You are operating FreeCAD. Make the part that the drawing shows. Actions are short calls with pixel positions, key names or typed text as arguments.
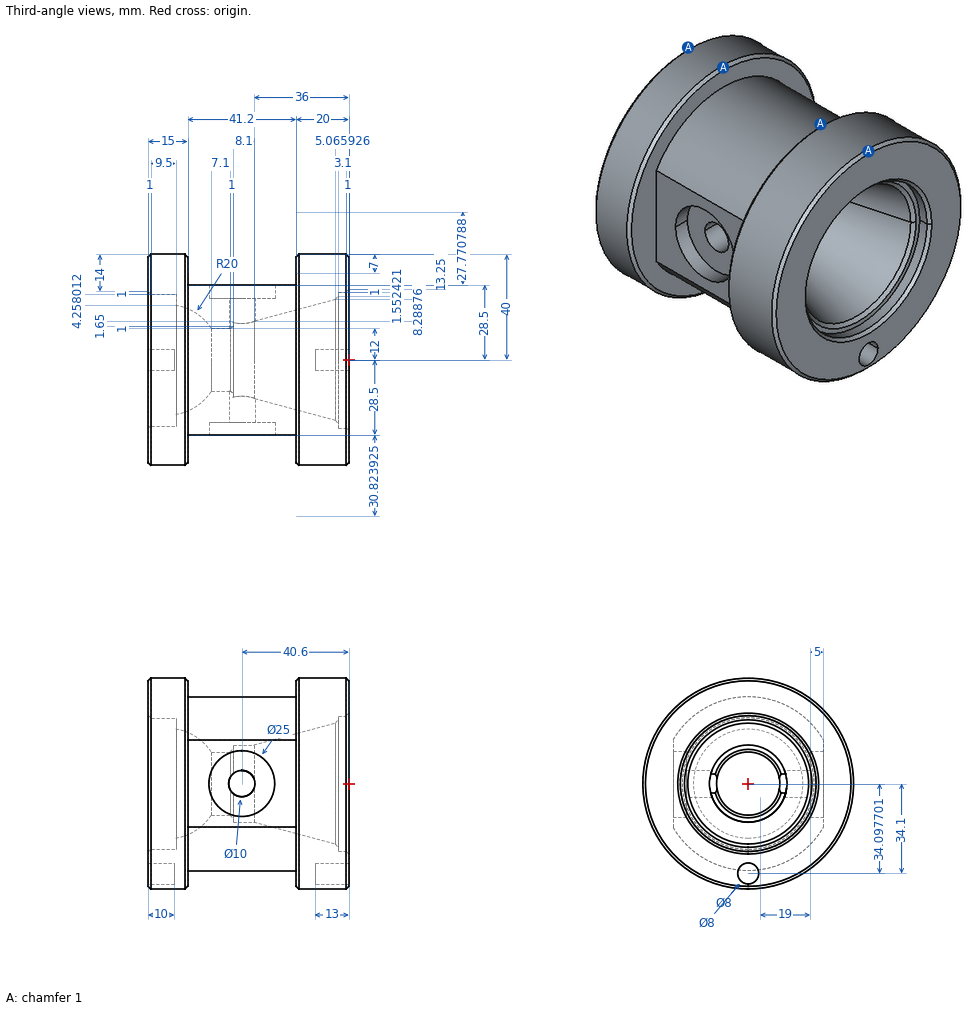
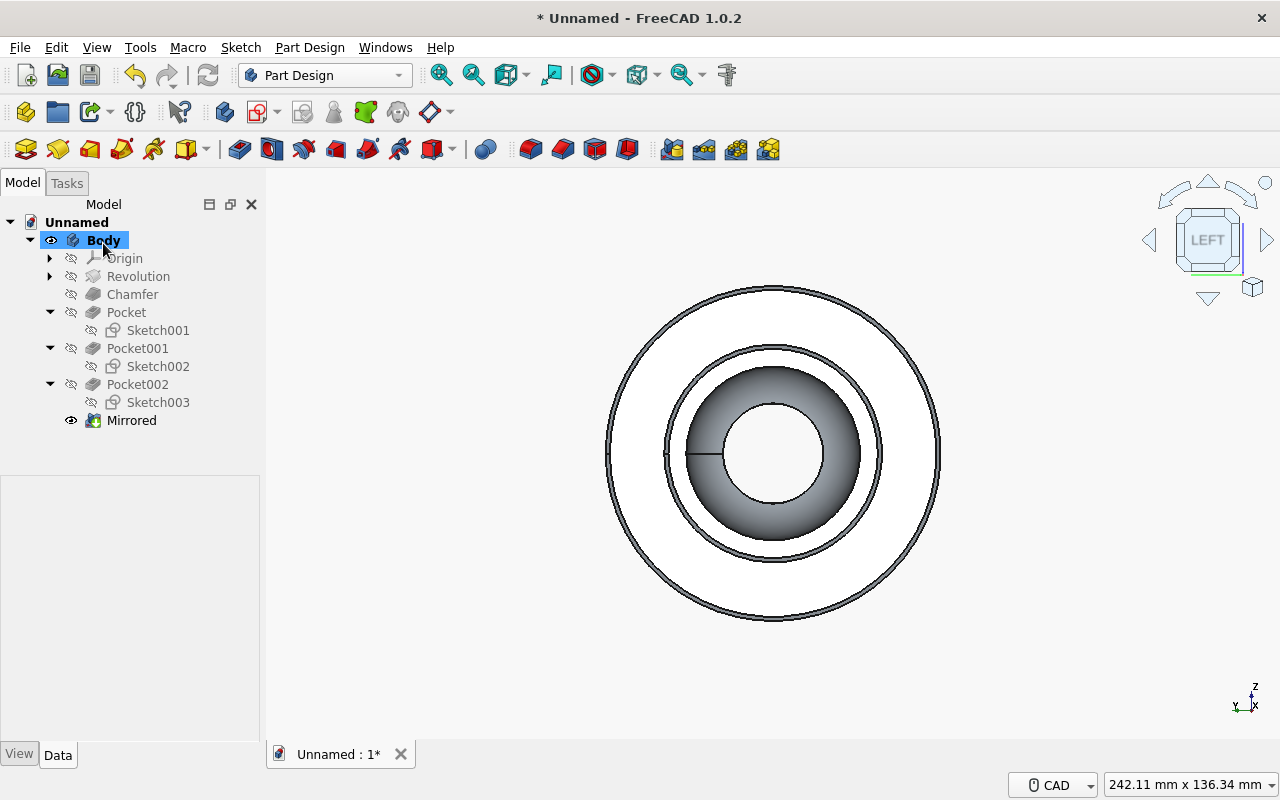
click(633, 453)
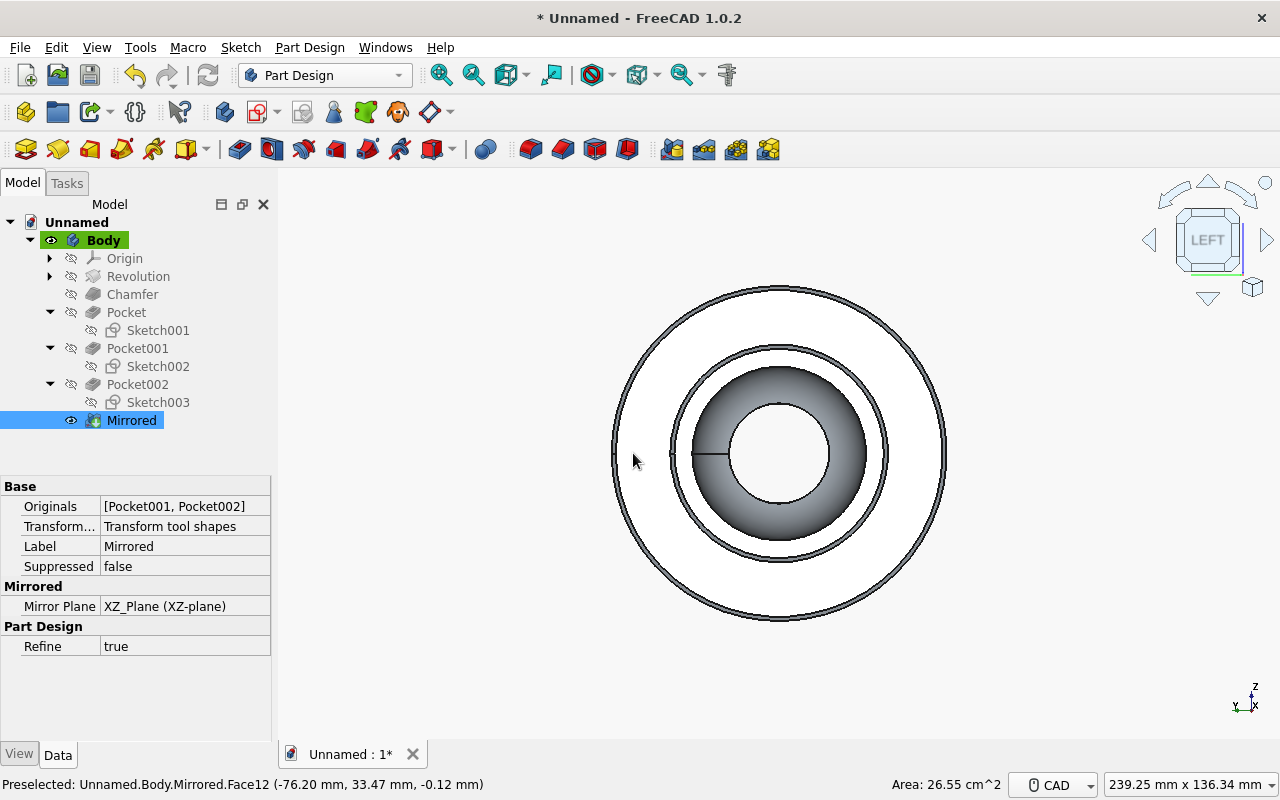
click(258, 112)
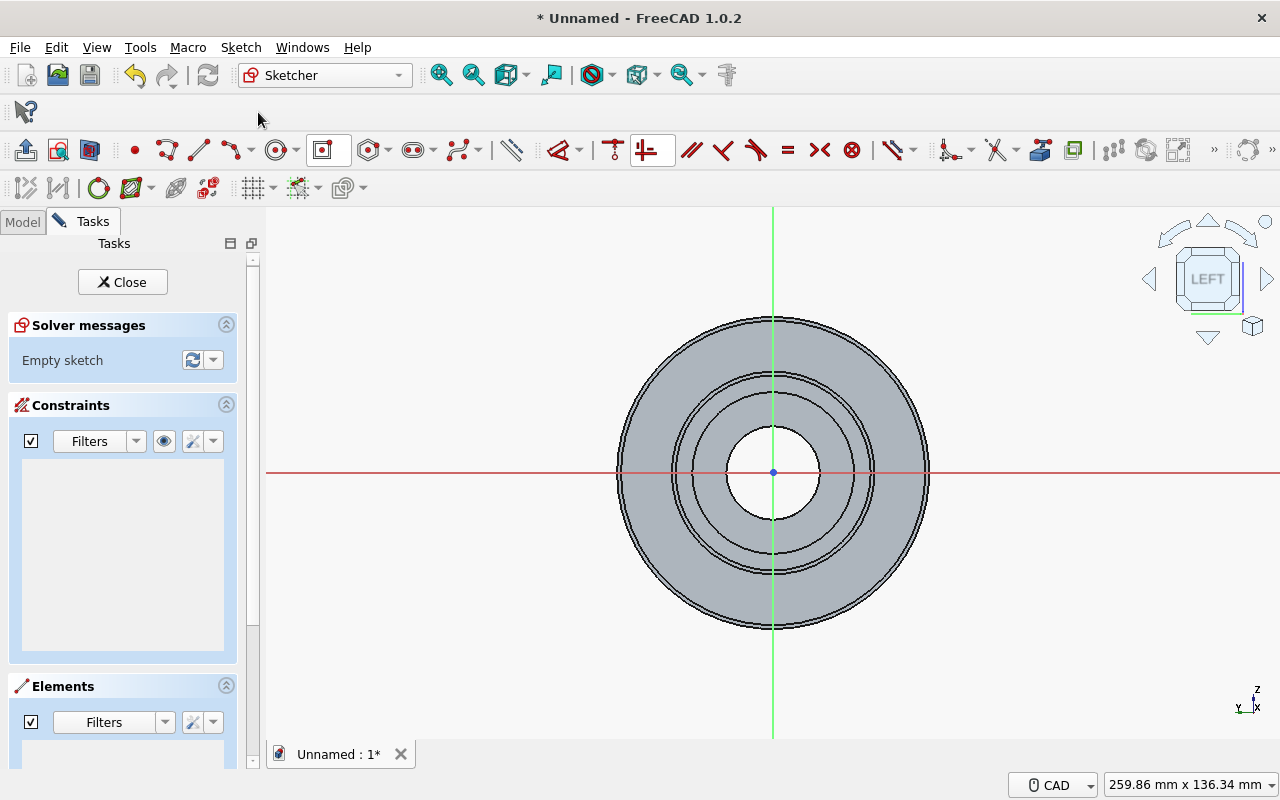
scroll(780, 619, up, 12)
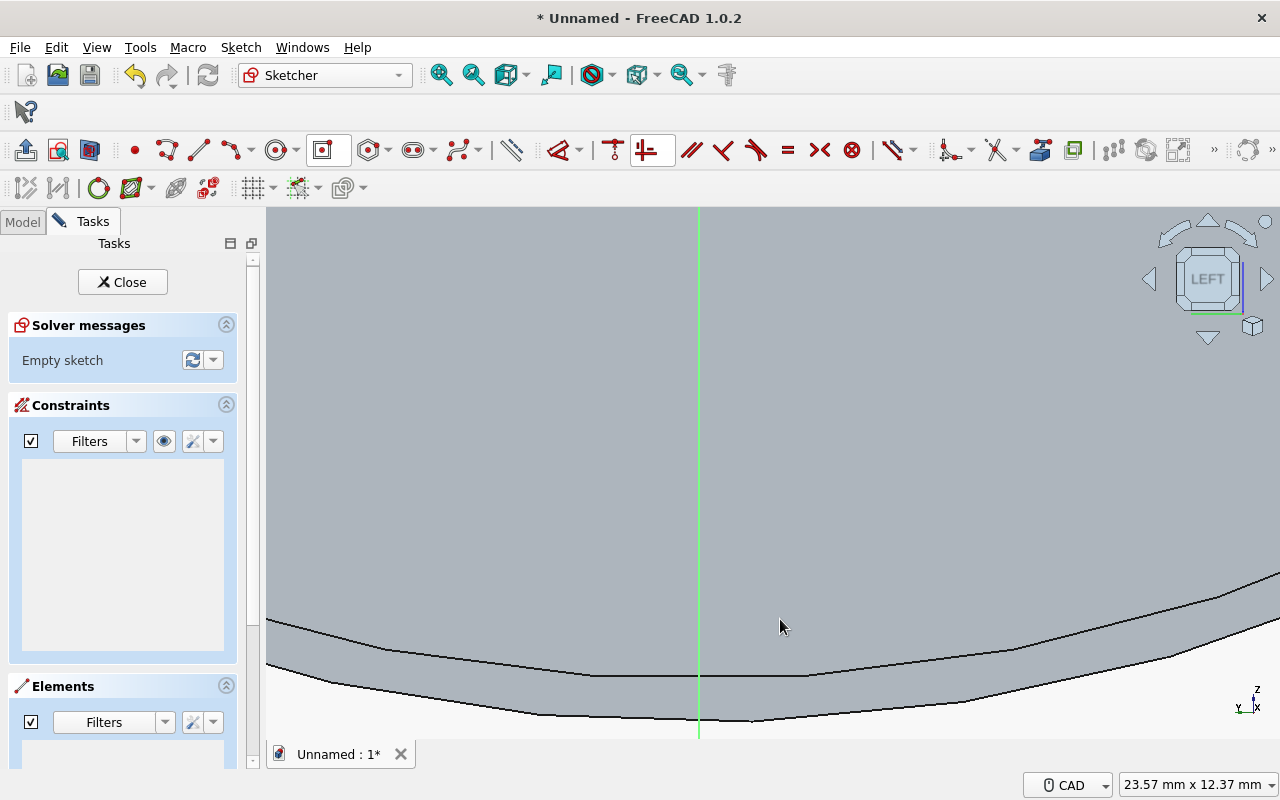
click(276, 150)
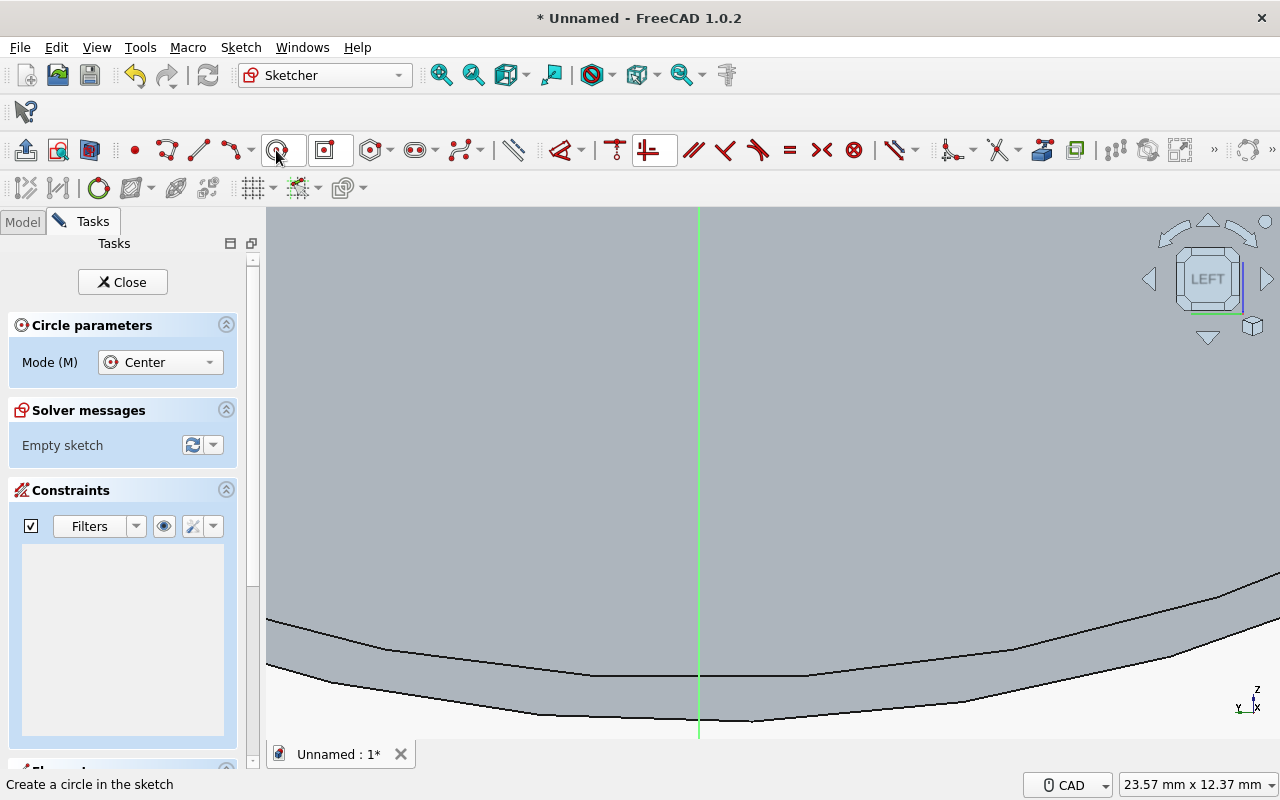
click(699, 468)
move(821, 347)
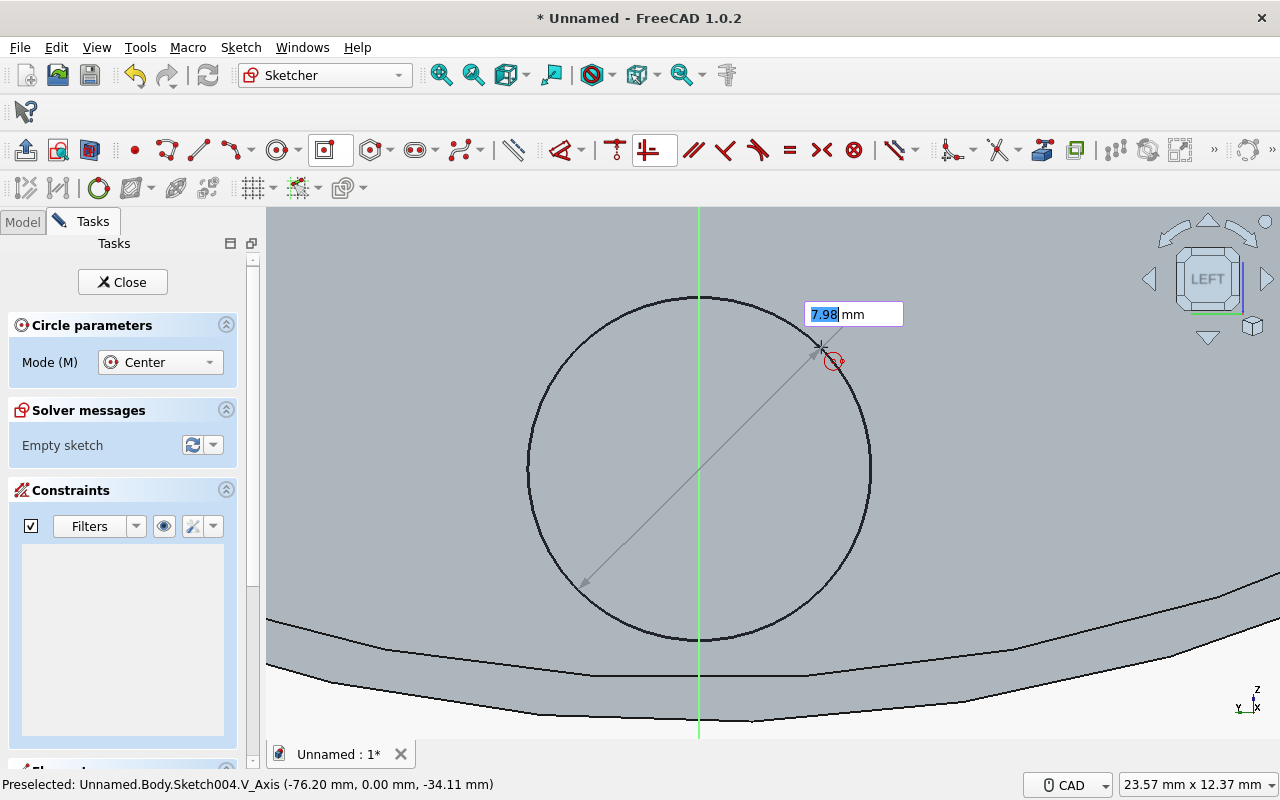
text(8)
key(Return)
key(Escape)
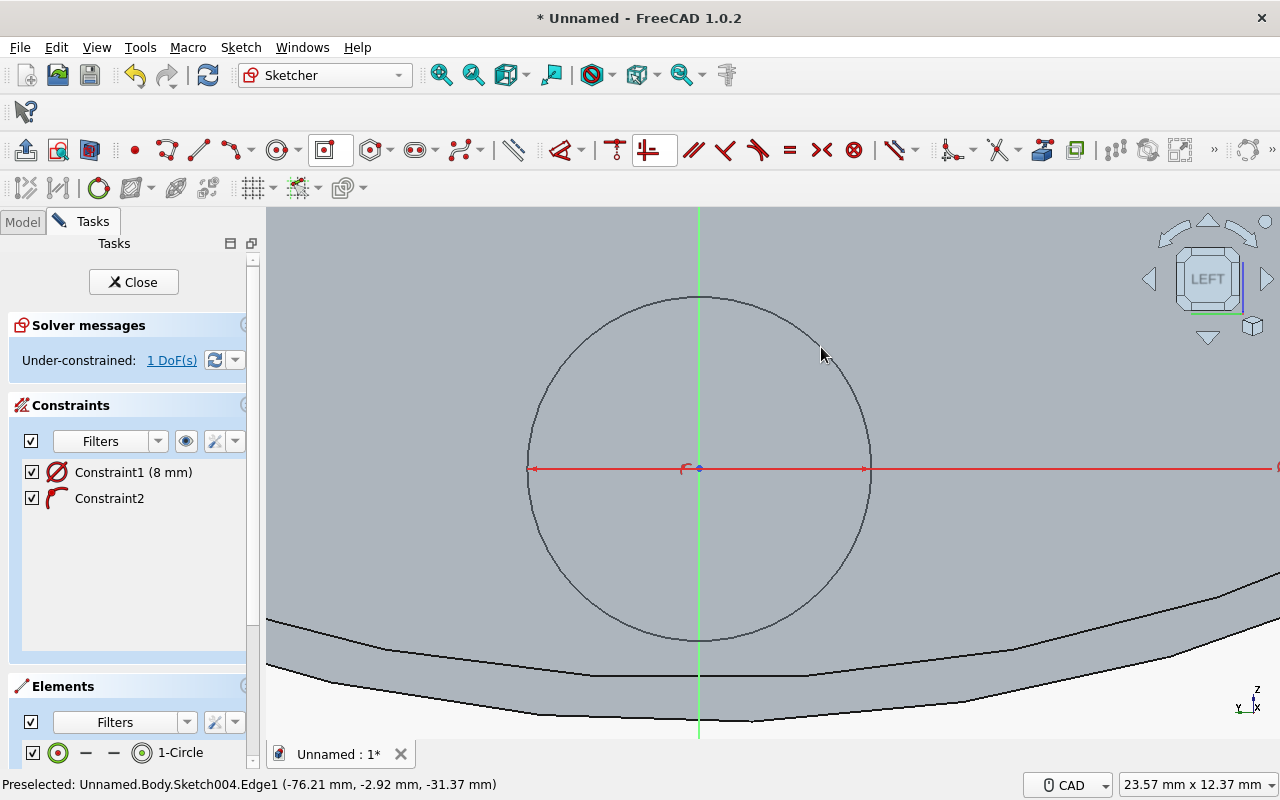
click(560, 150)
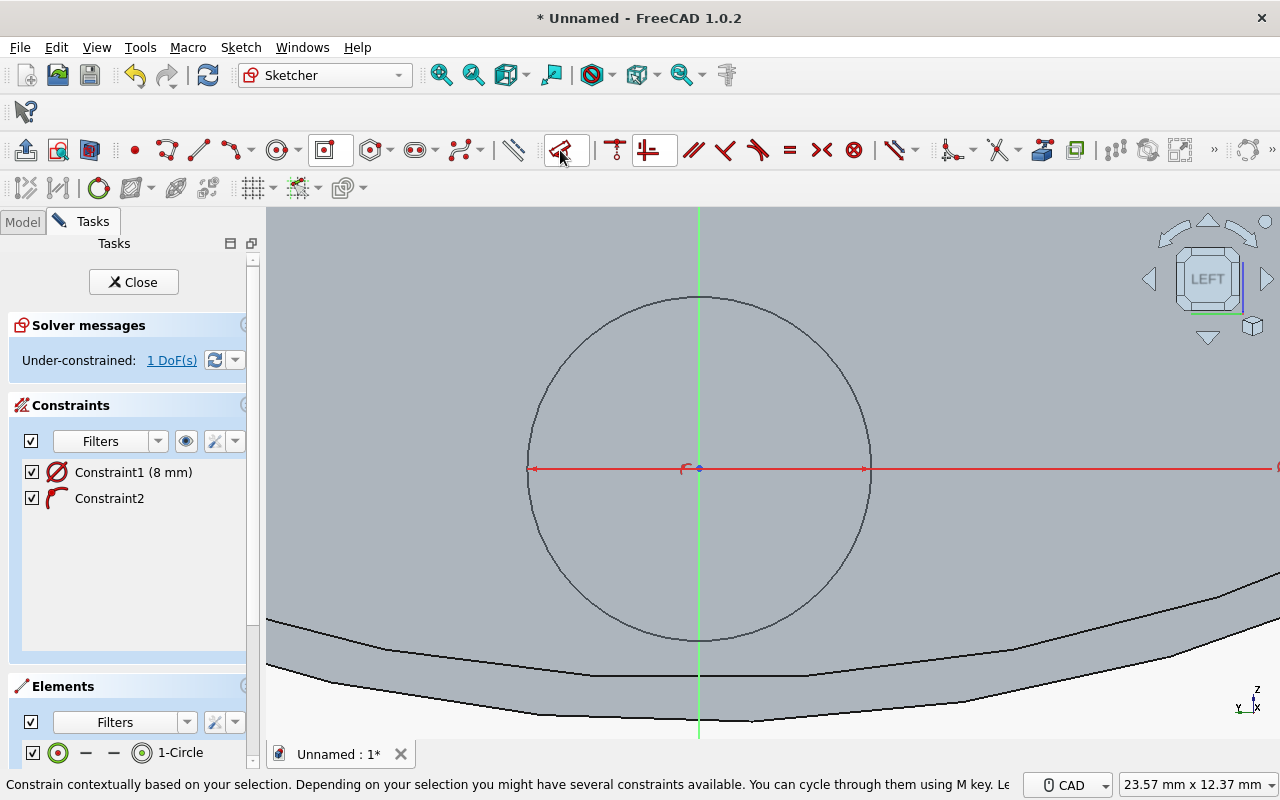
click(699, 469)
click(733, 352)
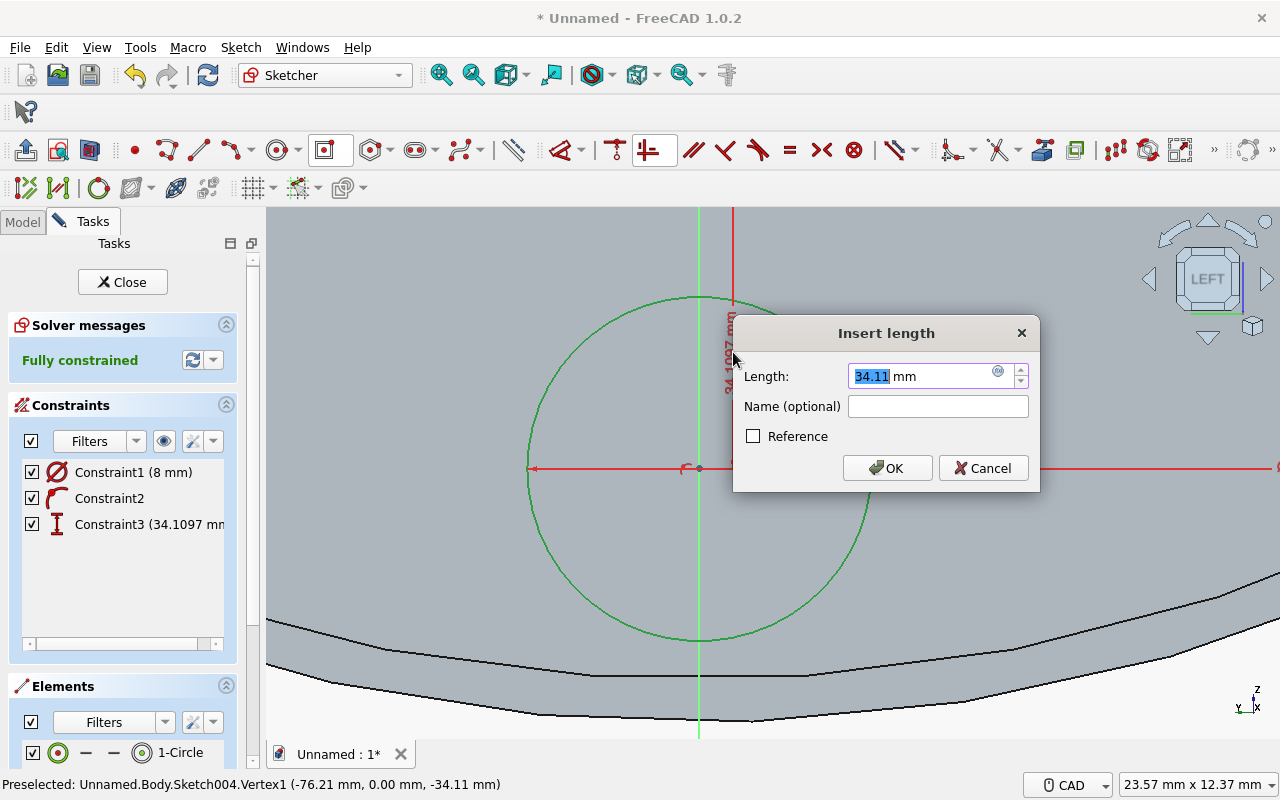
text(34.097701)
key(Return)
key(Escape)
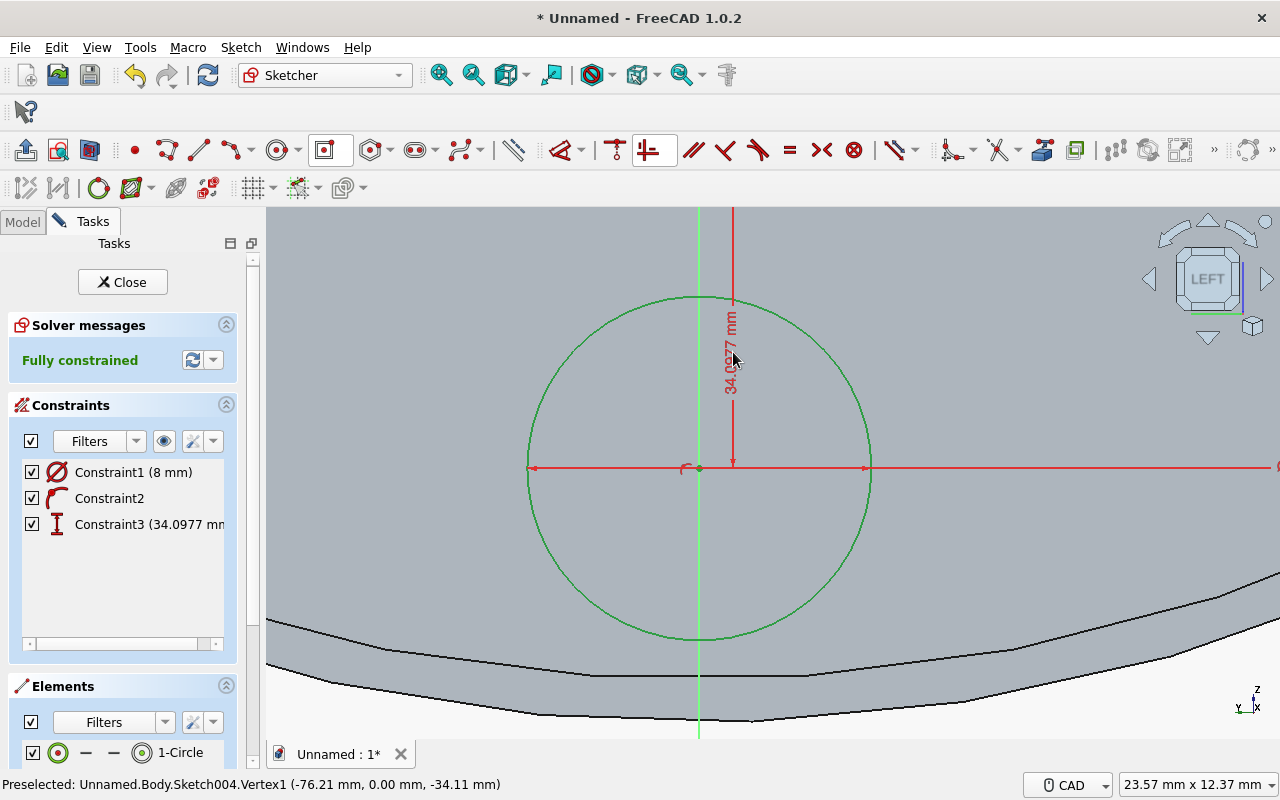
click(123, 282)